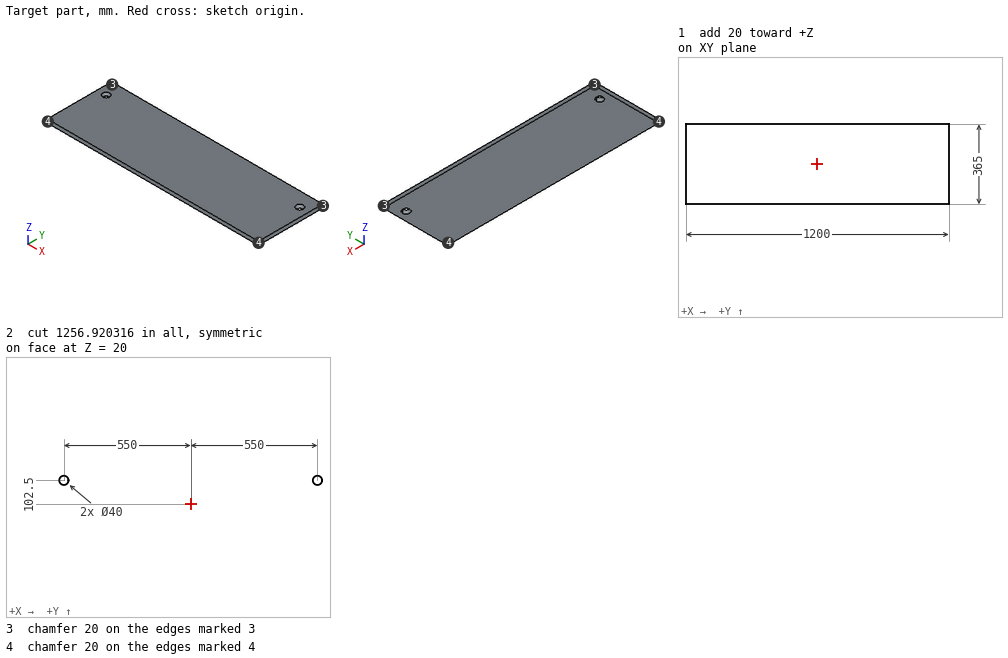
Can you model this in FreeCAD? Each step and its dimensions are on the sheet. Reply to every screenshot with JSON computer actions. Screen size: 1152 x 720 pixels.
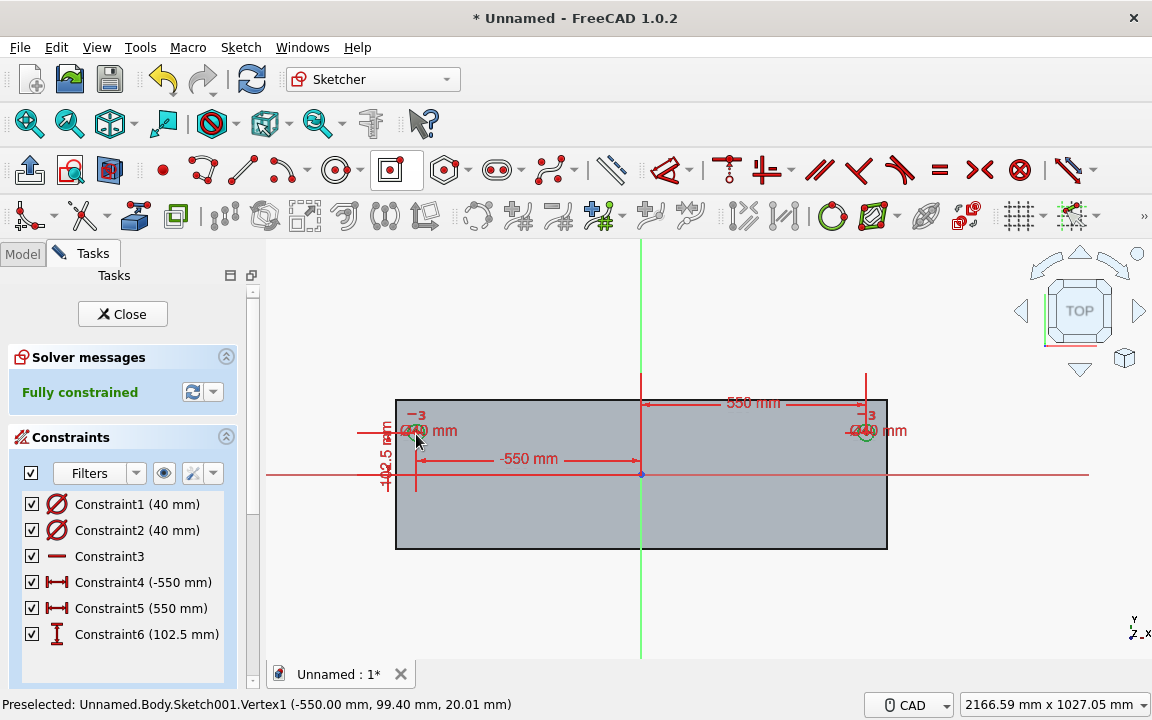
{"action": "left_click", "coordinate": [123, 314]}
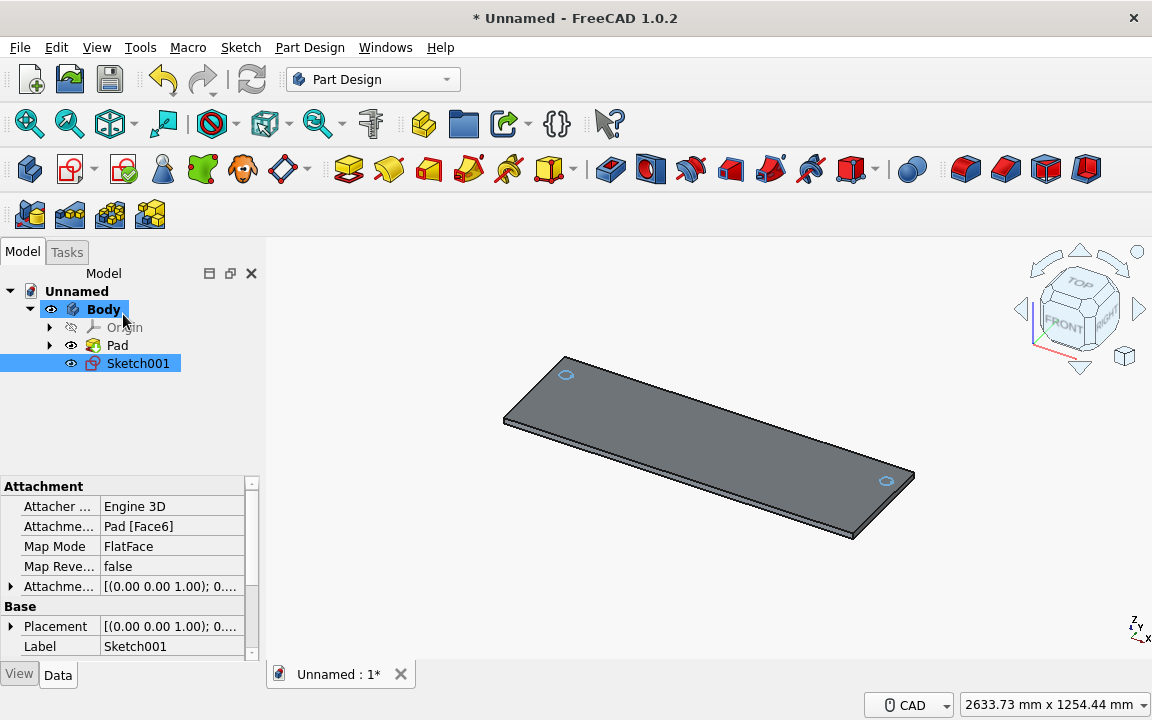
{"action": "left_click", "coordinate": [612, 170]}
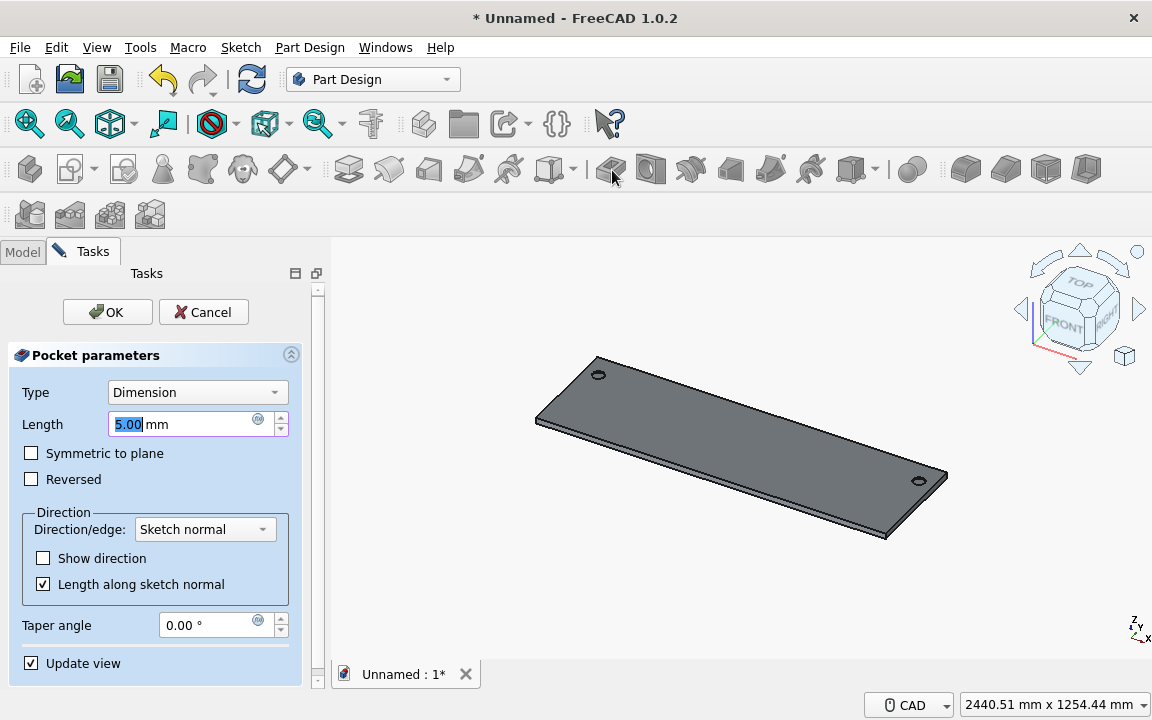
{"action": "type", "text": "1256.920316"}
{"action": "key", "text": "Tab"}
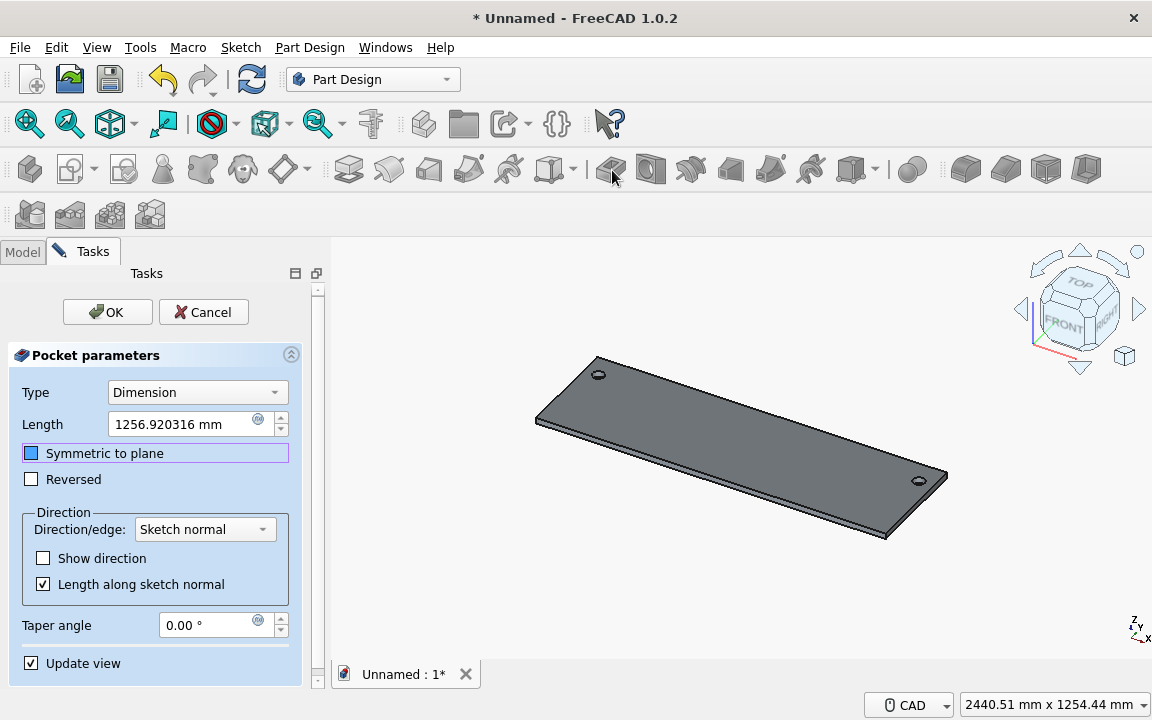
{"action": "left_click", "coordinate": [30, 453]}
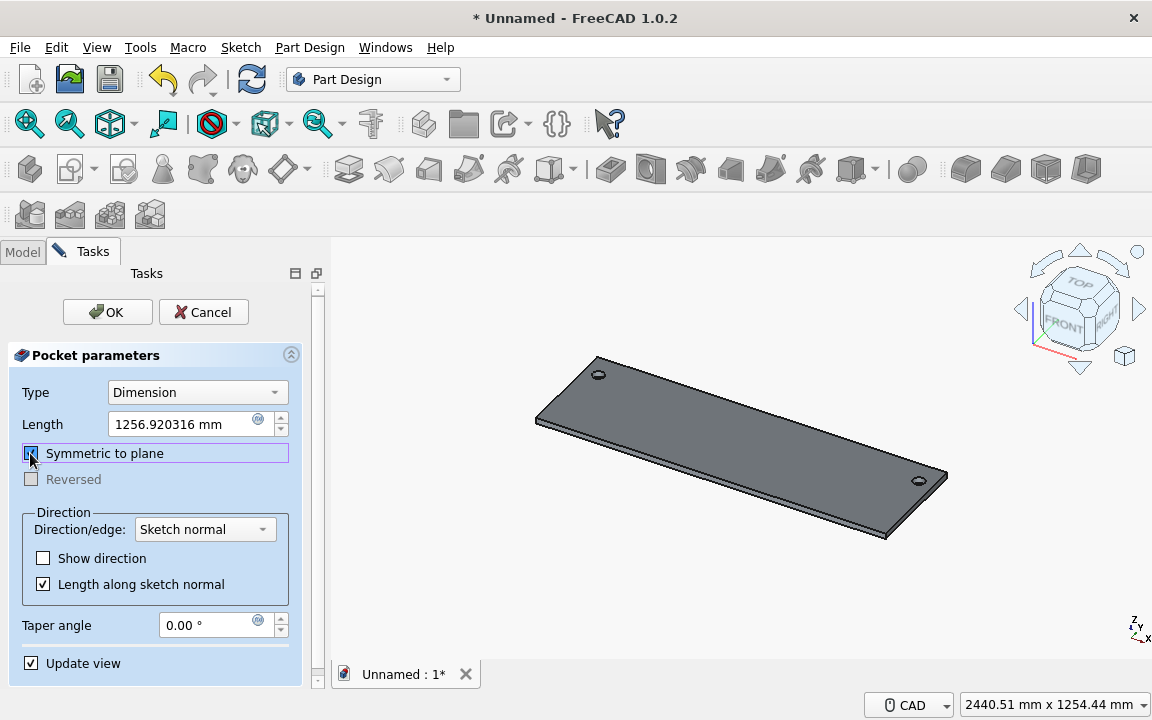
{"action": "left_click", "coordinate": [108, 312]}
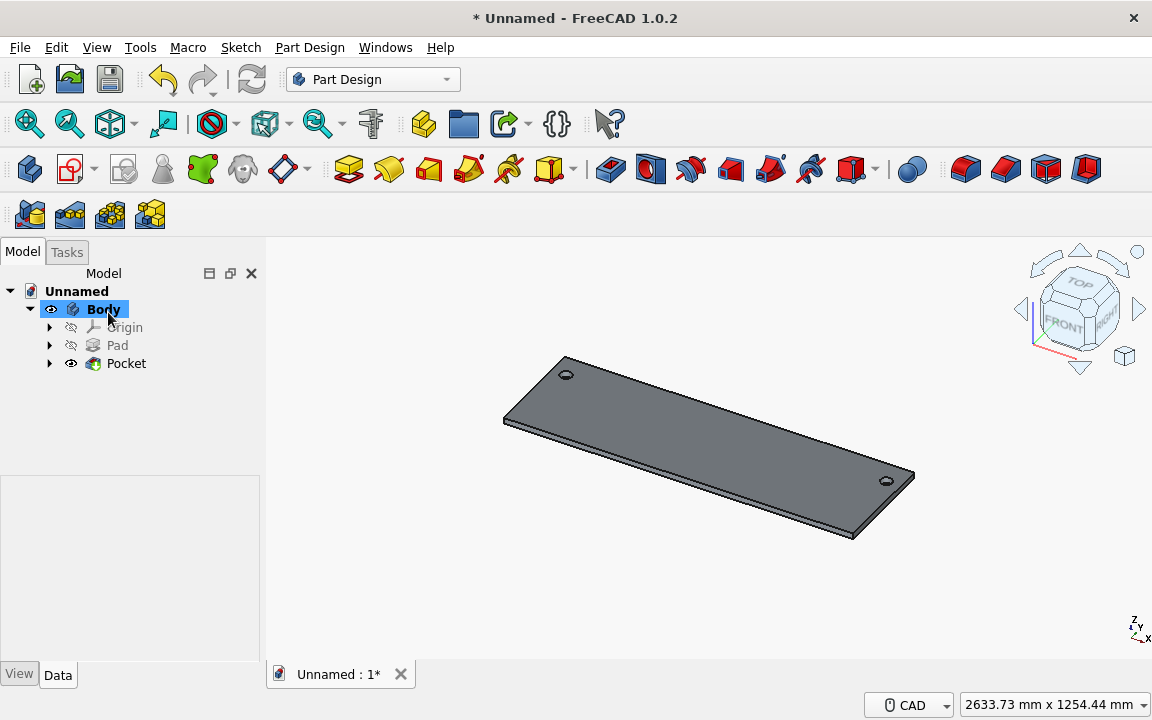
{"action": "scroll", "coordinate": [565, 359], "scroll_direction": "up", "scroll_amount": 9}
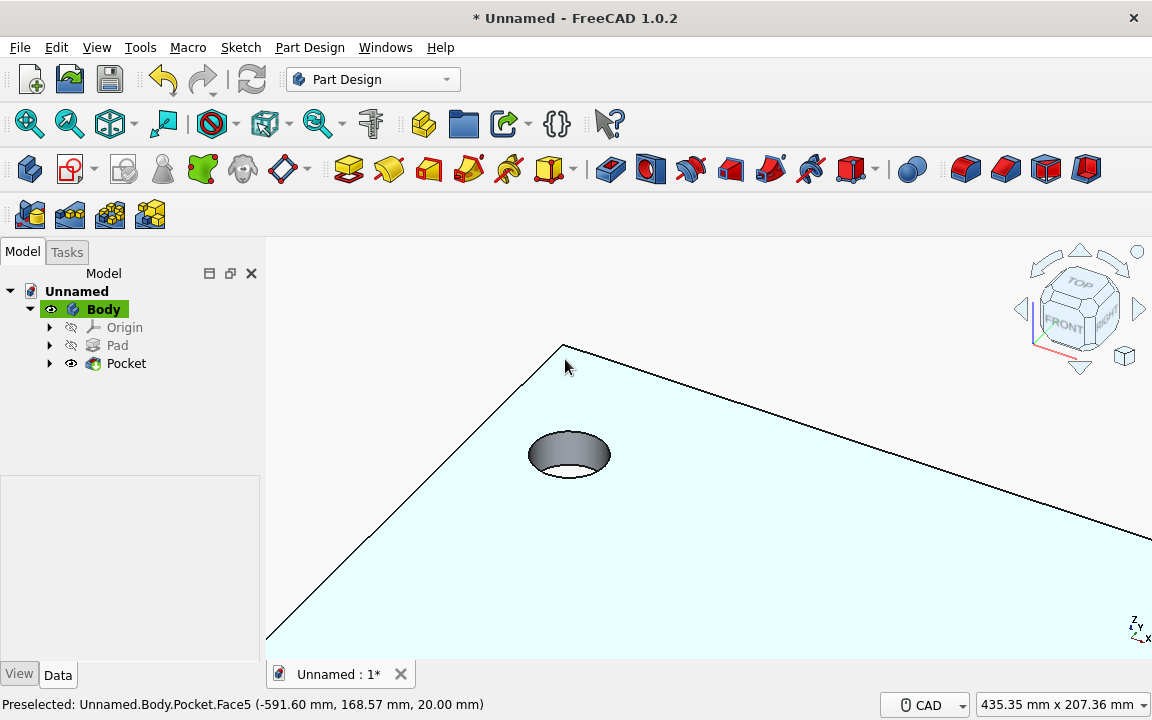
{"action": "left_click", "coordinate": [30, 124]}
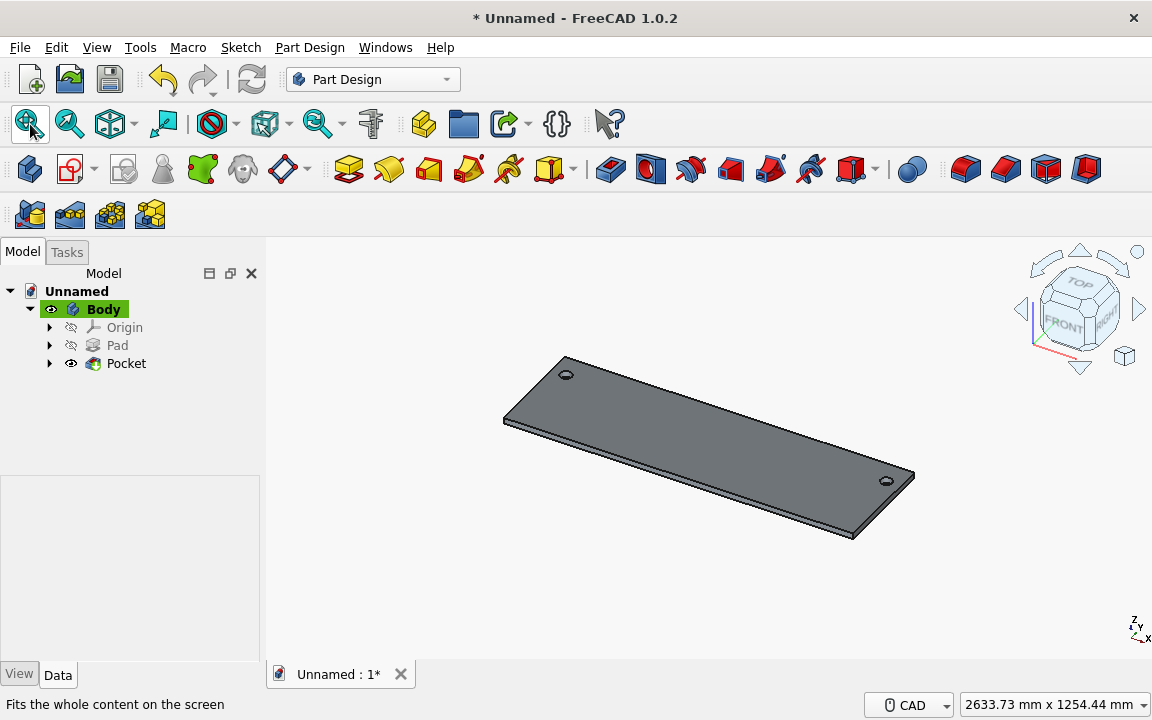
{"action": "key", "text": "0"}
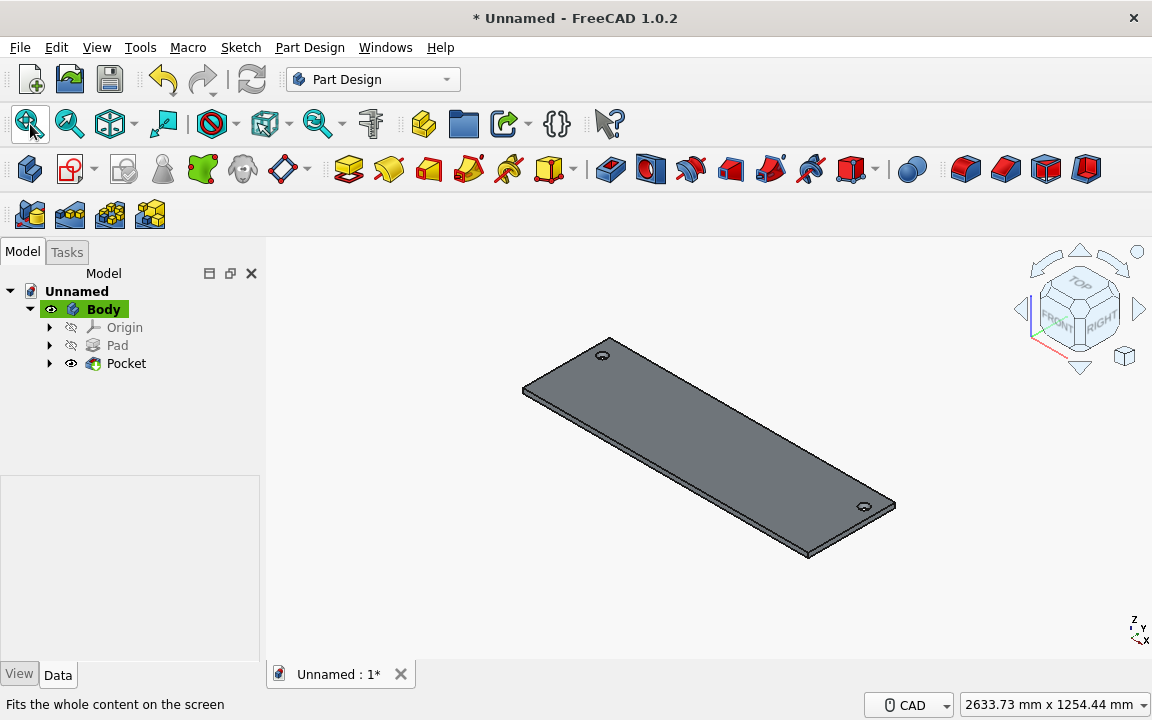
{"action": "scroll", "coordinate": [610, 340], "scroll_direction": "up", "scroll_amount": 9}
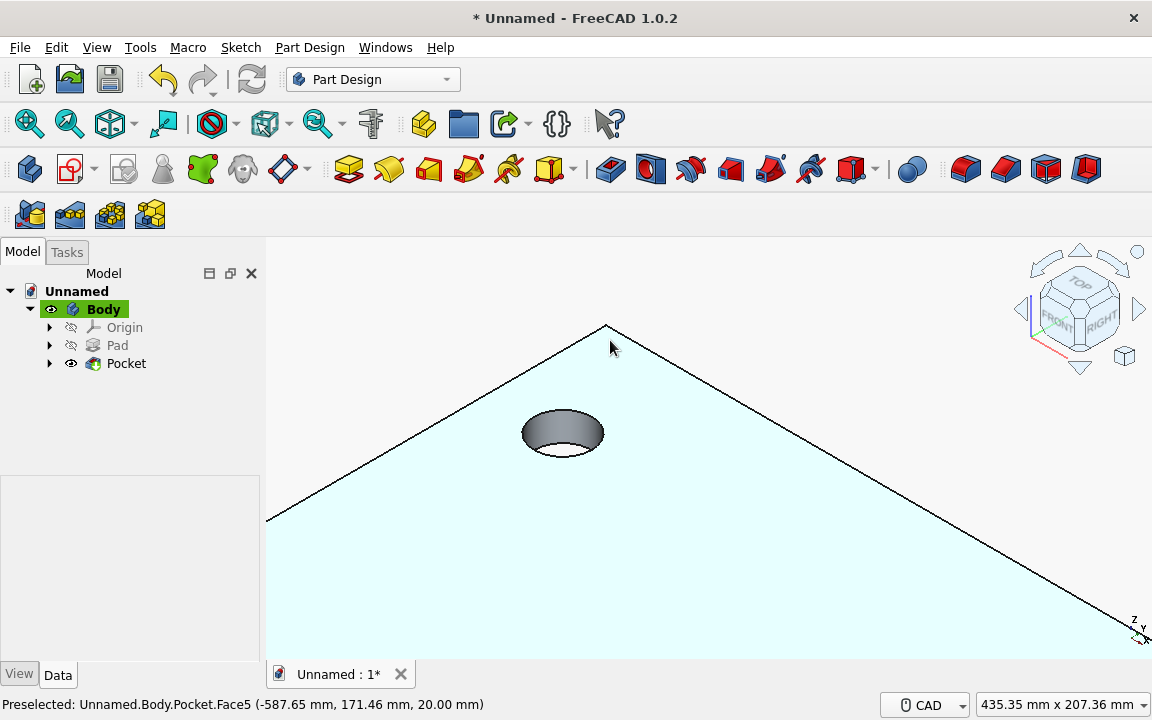
{"action": "key", "text": "v f"}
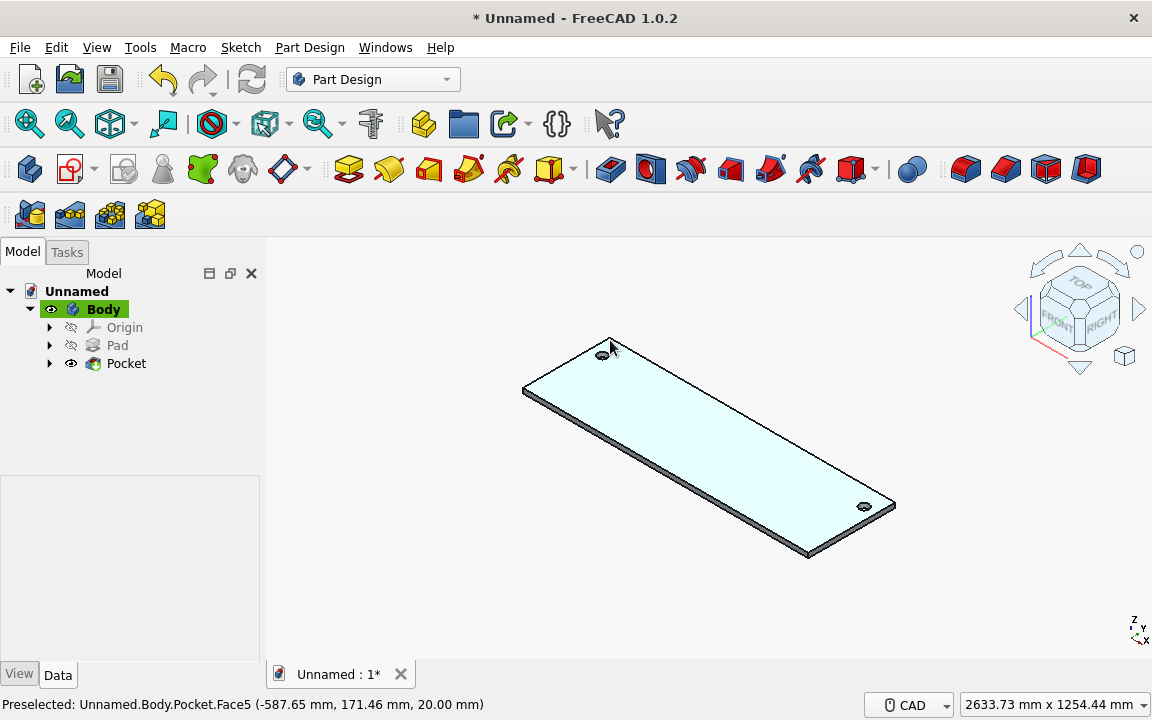
{"action": "key", "text": "2"}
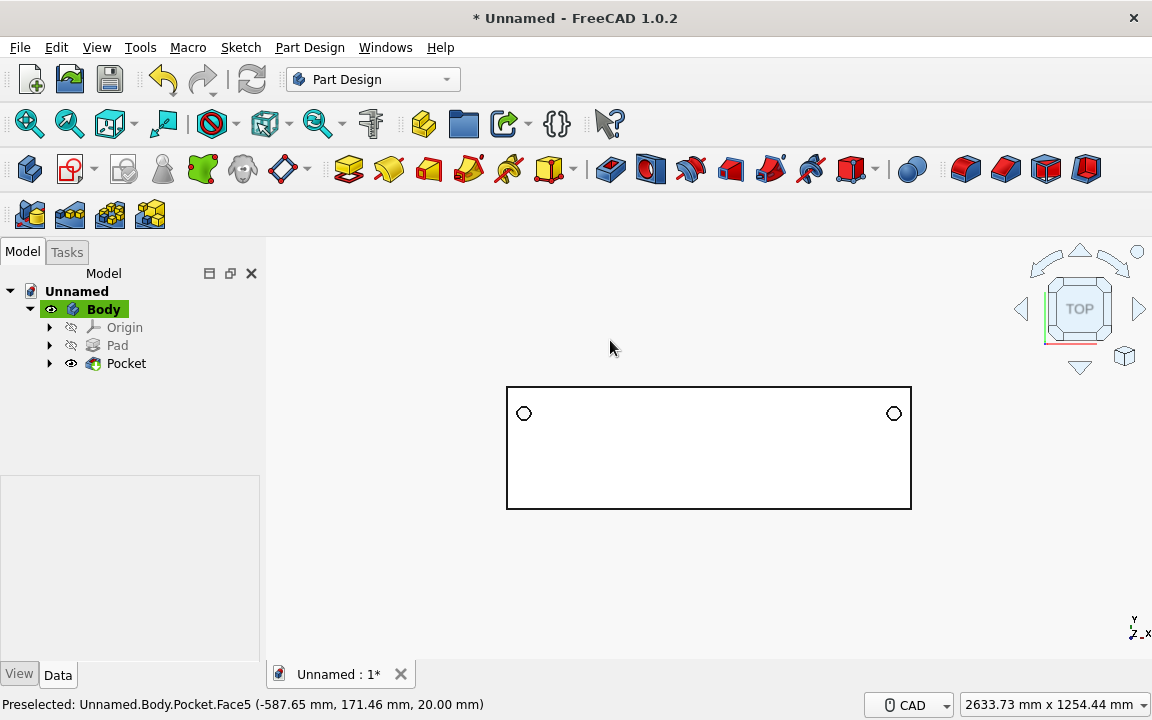
{"action": "scroll", "coordinate": [507, 386], "scroll_direction": "up", "scroll_amount": 9}